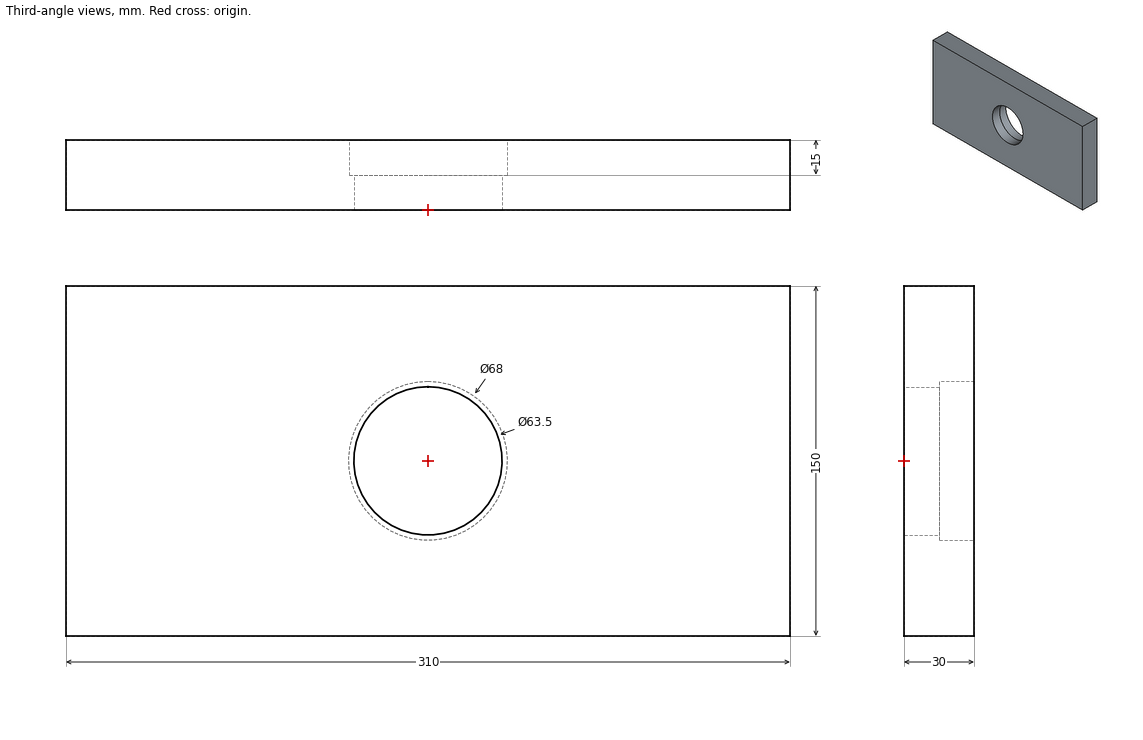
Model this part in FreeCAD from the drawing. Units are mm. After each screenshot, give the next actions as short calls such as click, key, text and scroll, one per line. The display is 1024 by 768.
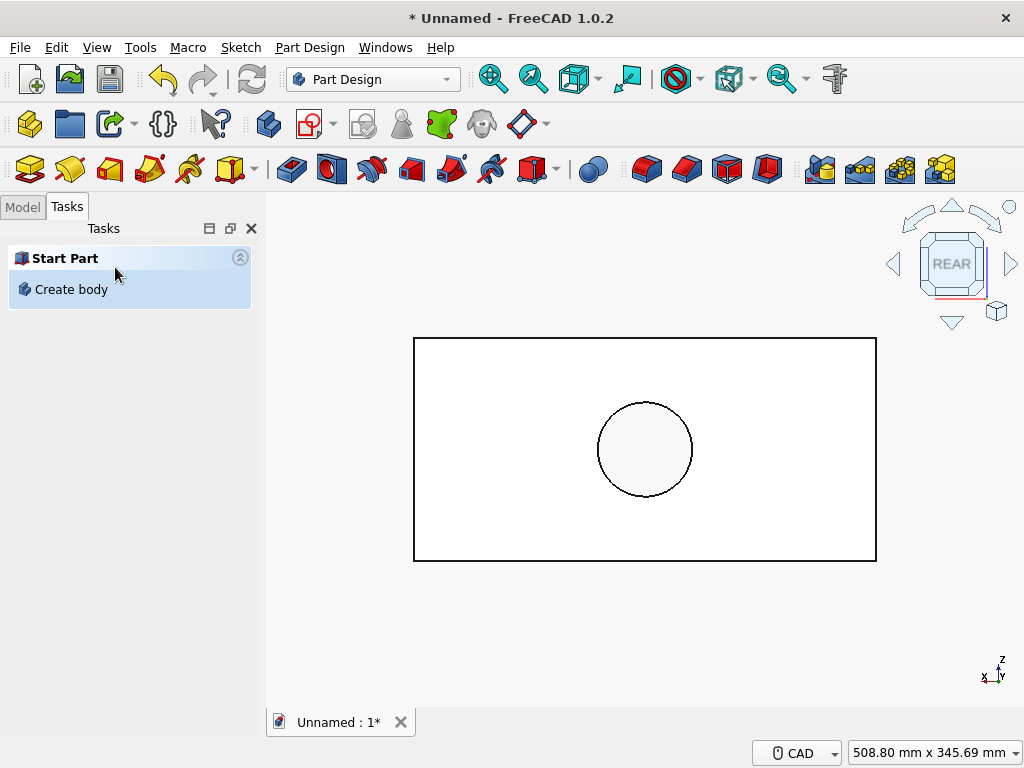
click(513, 448)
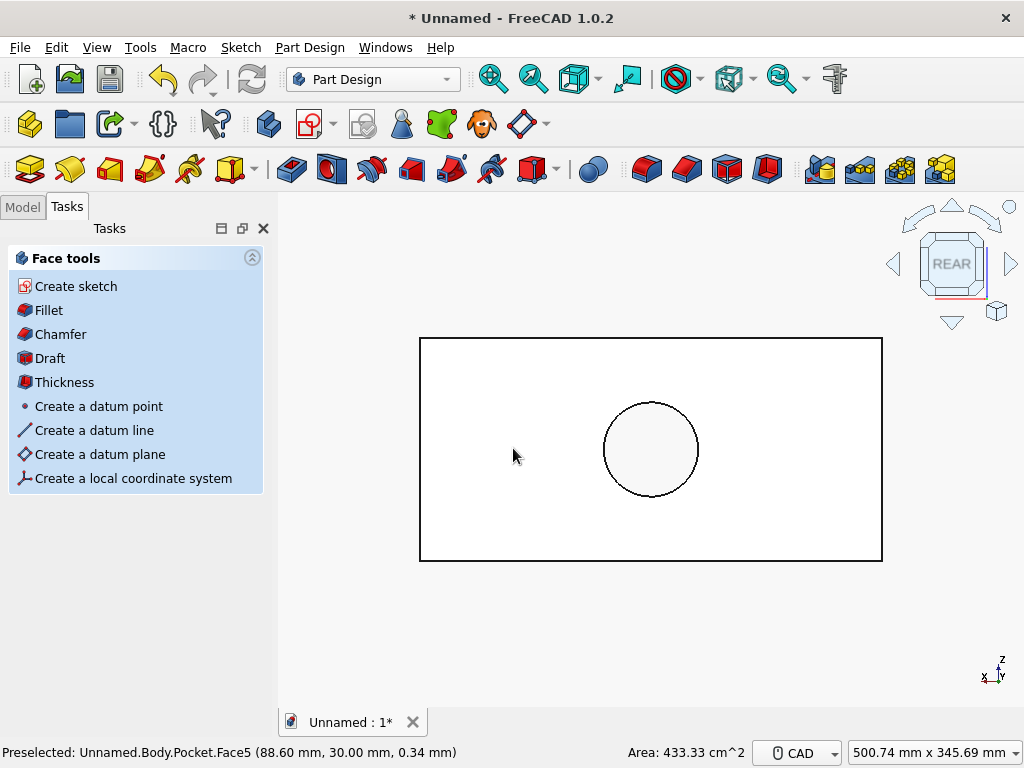
click(310, 124)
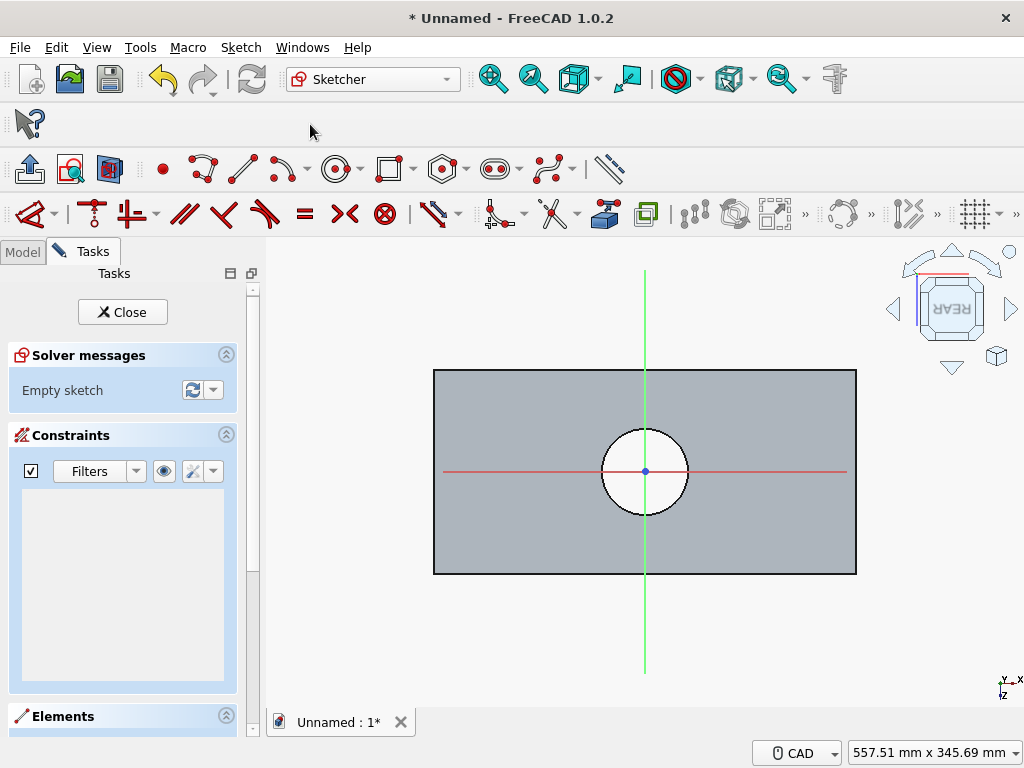
scroll(675, 472, up, 6)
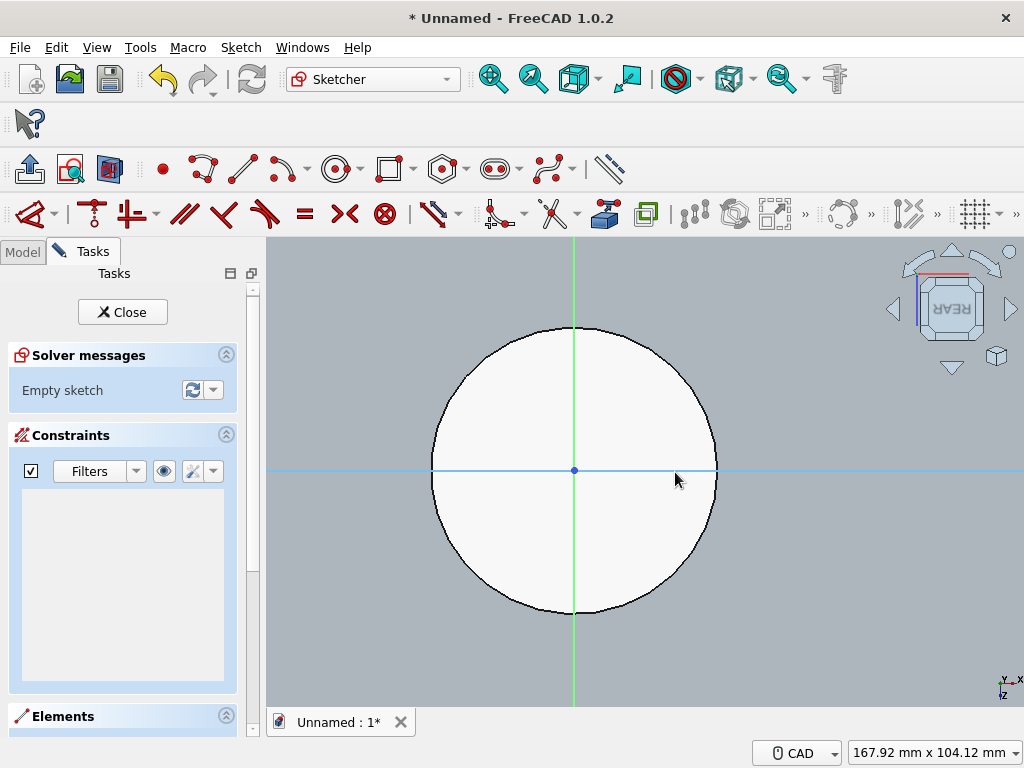
click(336, 170)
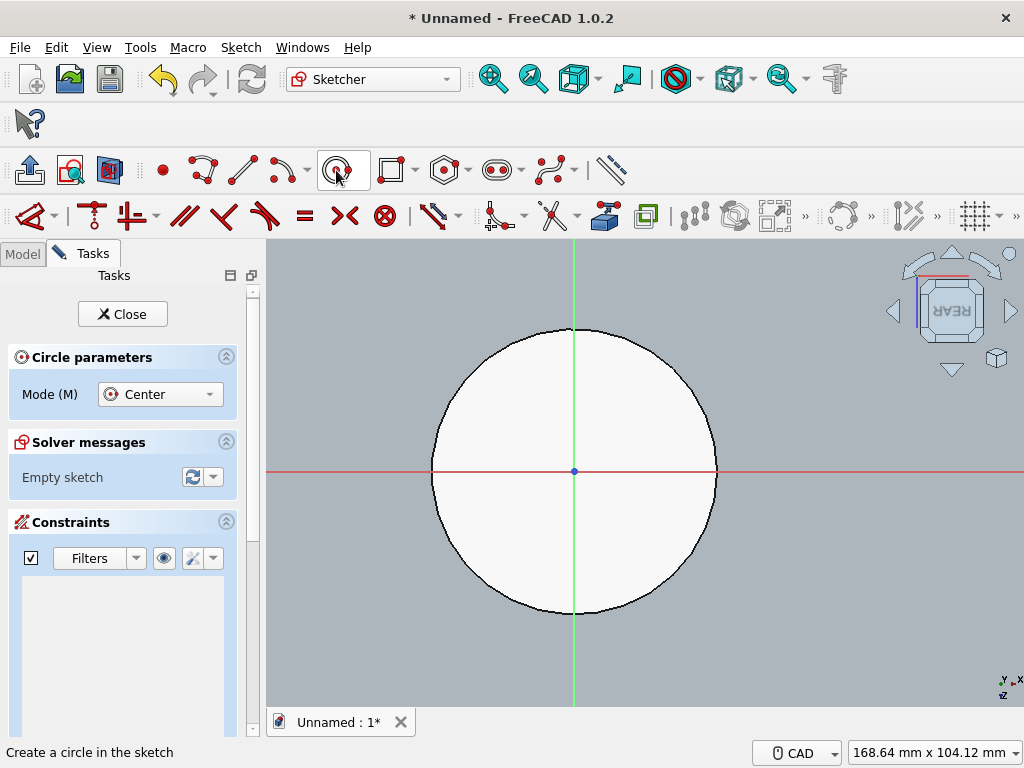
click(574, 472)
move(683, 364)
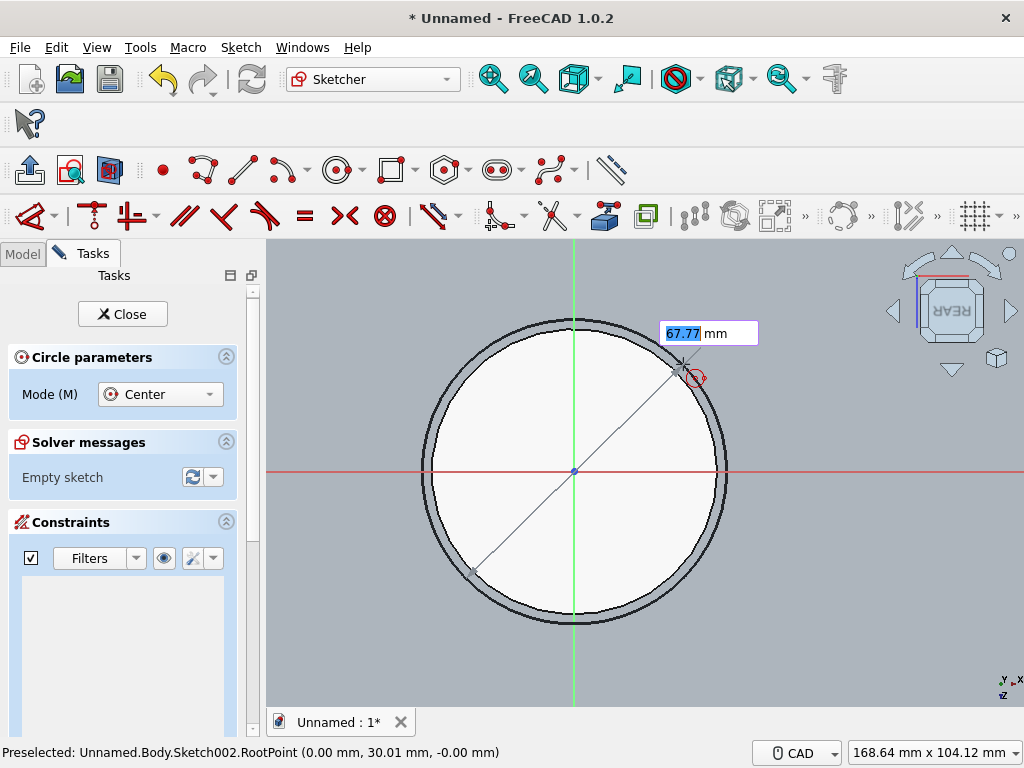
text(68)
key(Return)
key(Escape)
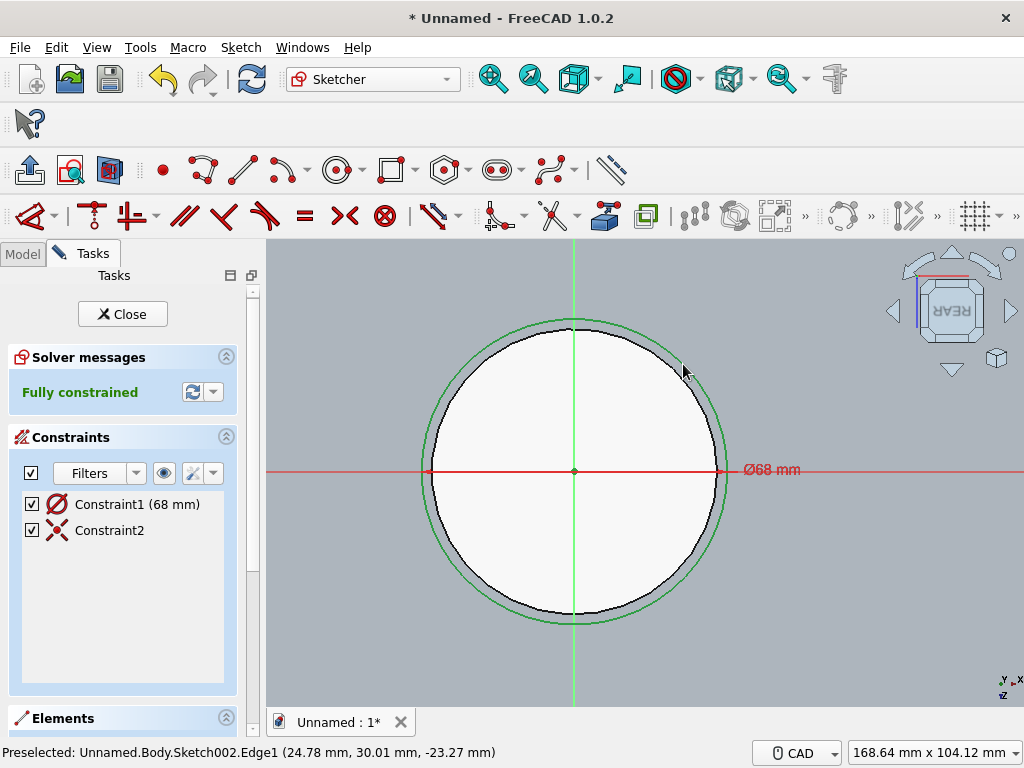
click(123, 314)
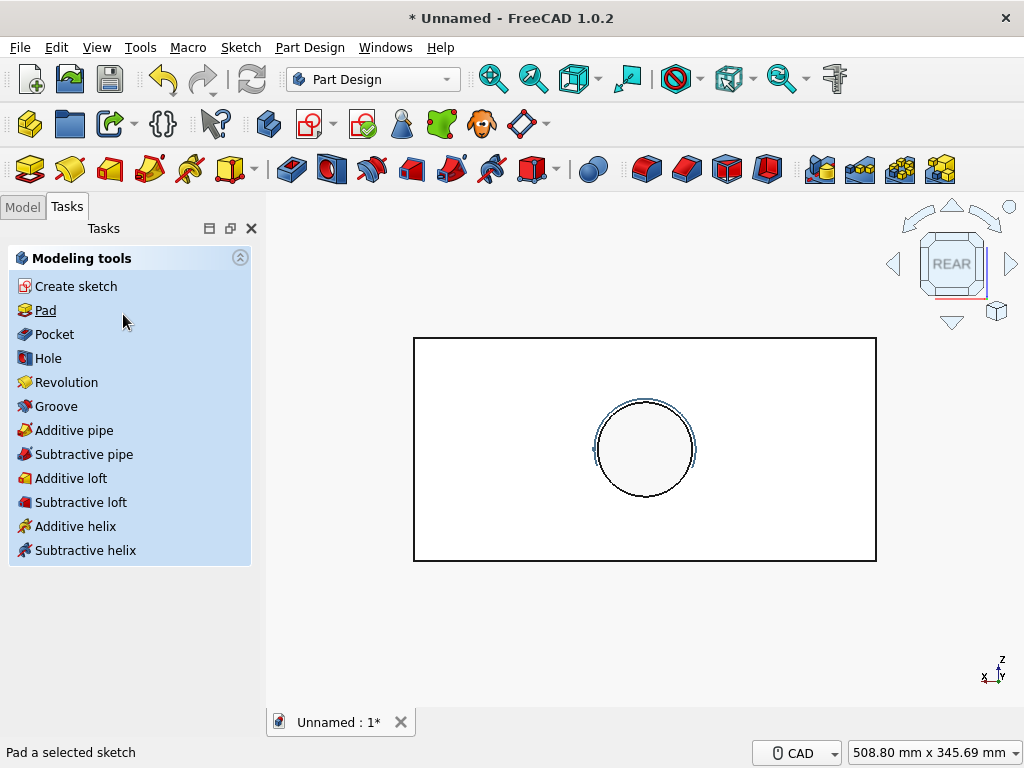
click(292, 170)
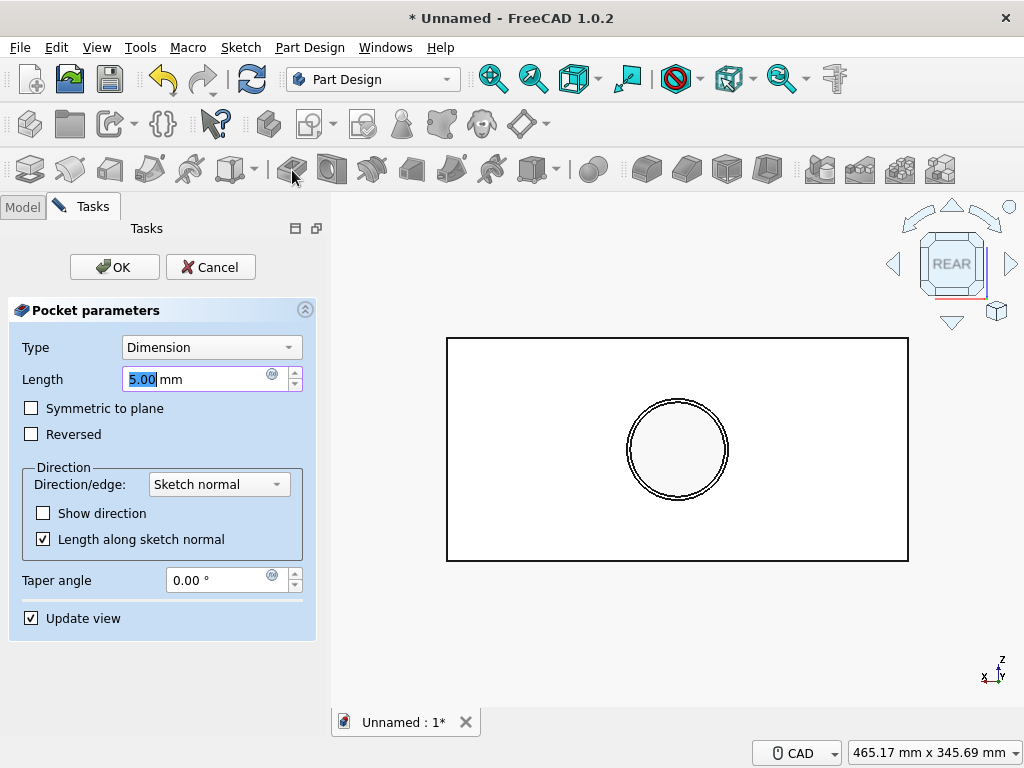
text(15)
key(Tab)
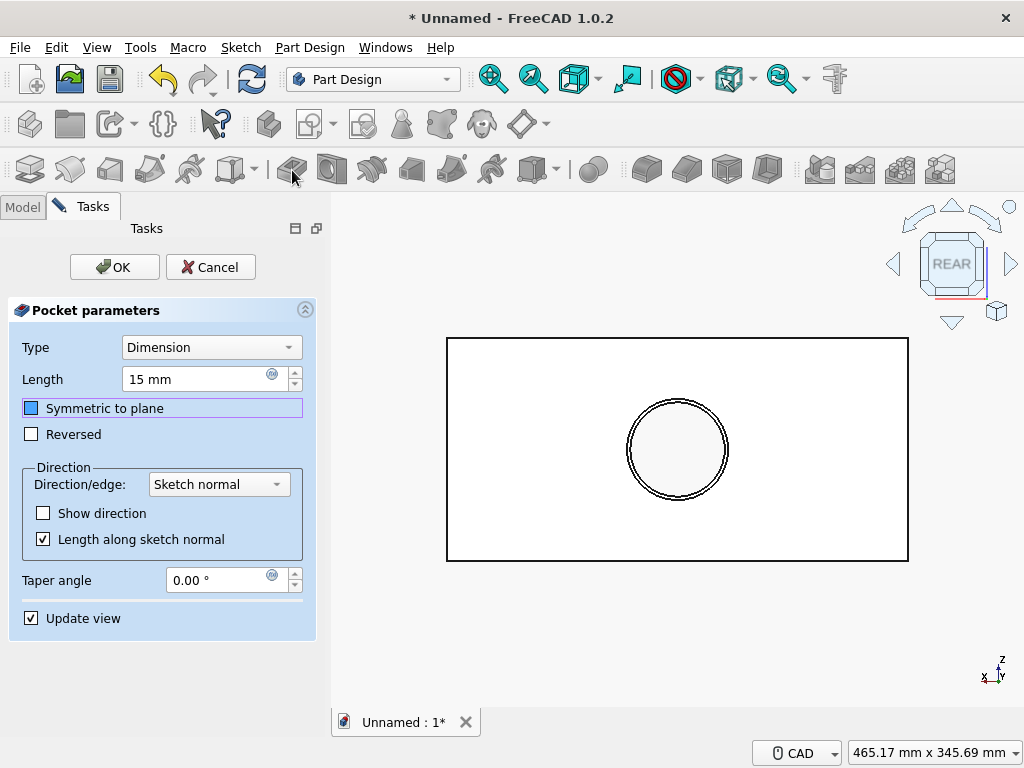
click(115, 267)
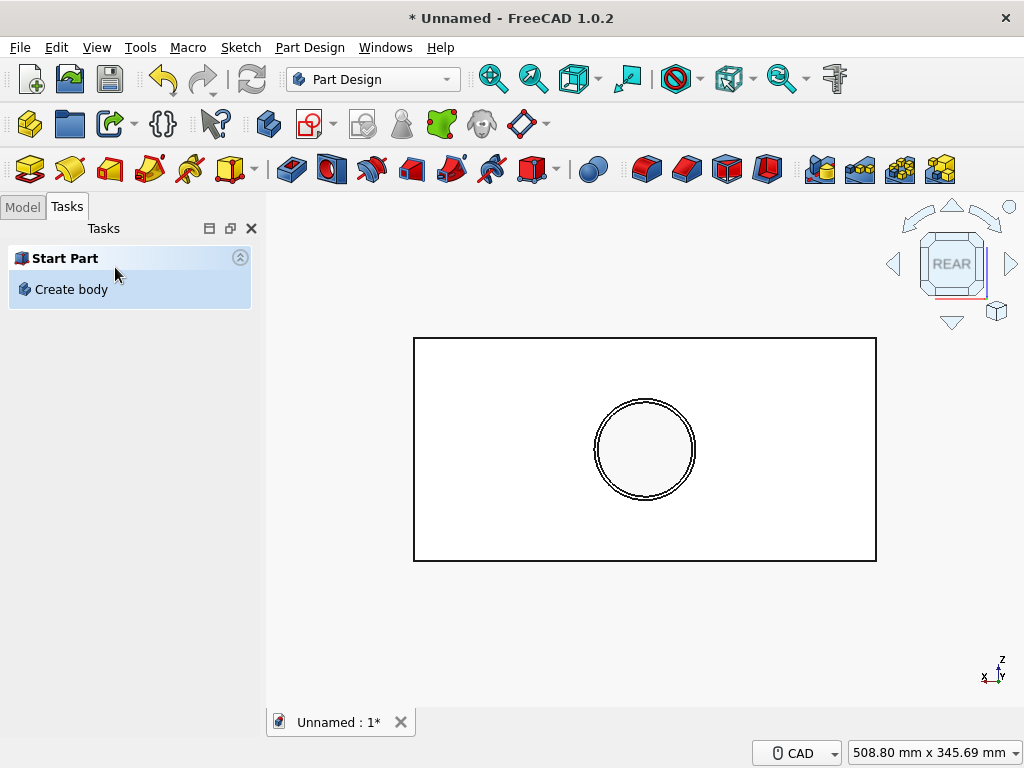
key(0)